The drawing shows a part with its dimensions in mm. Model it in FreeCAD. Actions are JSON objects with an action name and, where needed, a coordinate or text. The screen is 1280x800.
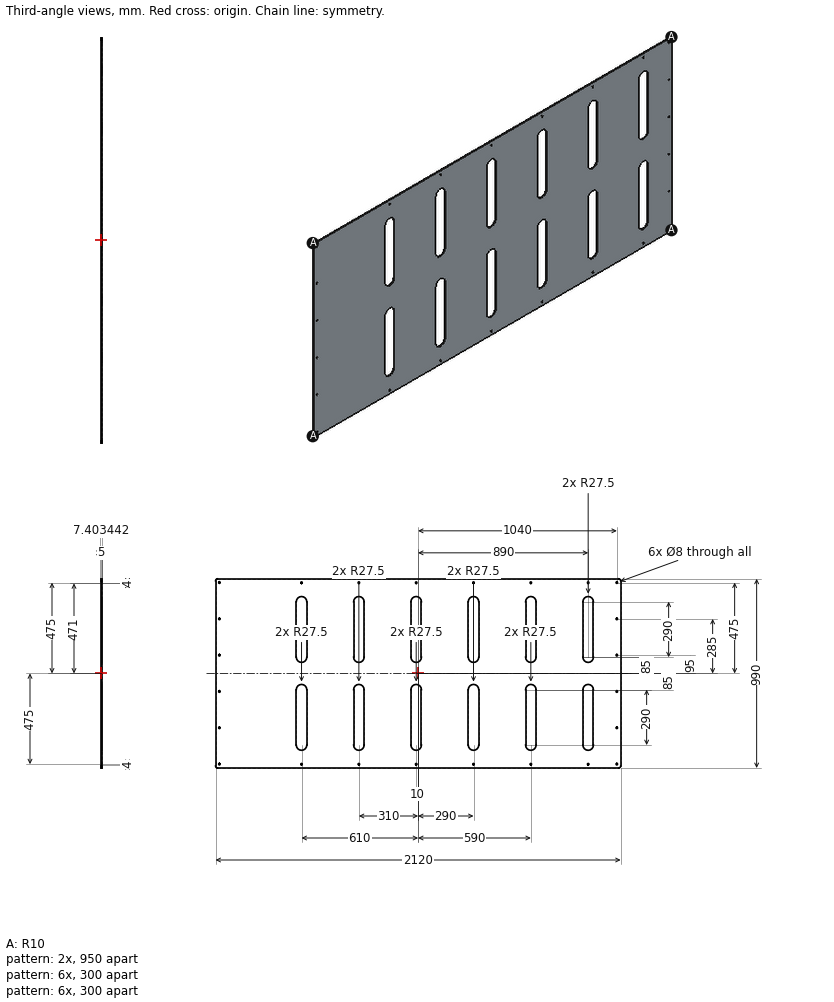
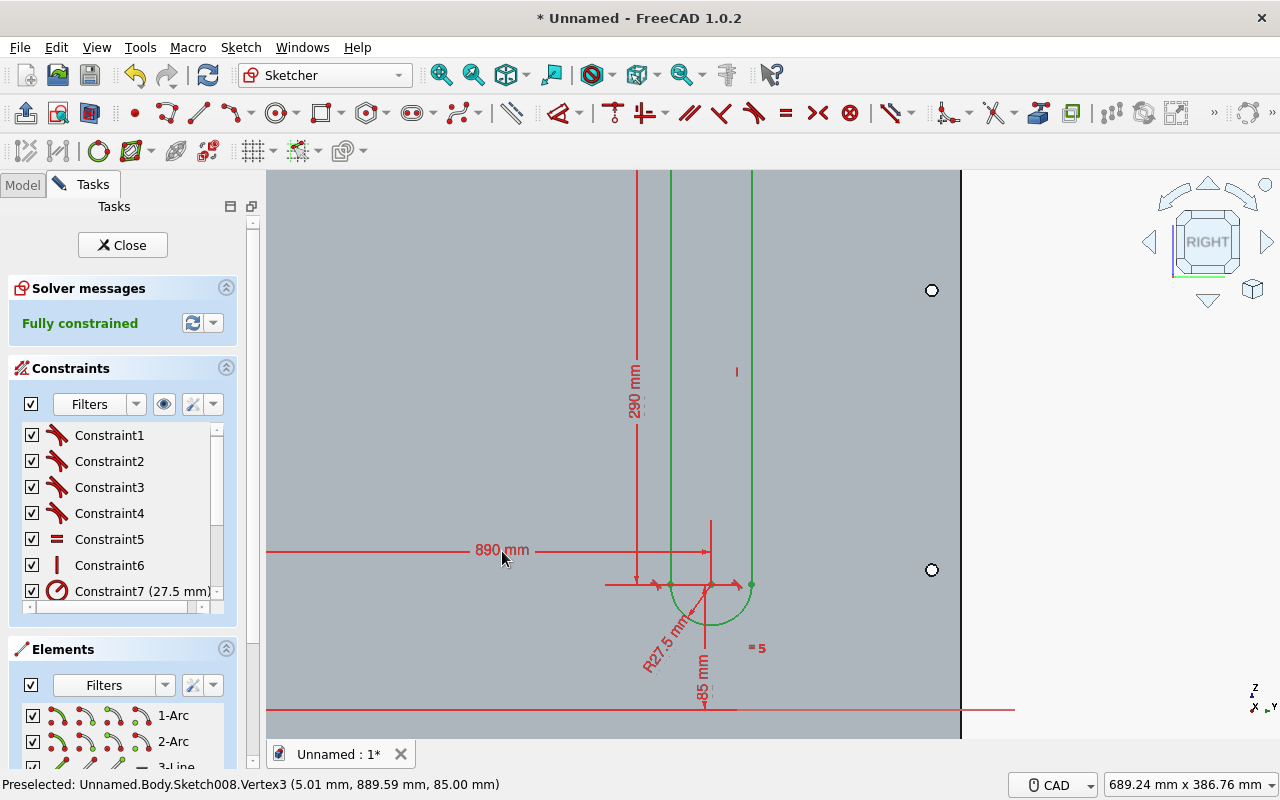
{"action": "left_click", "coordinate": [123, 245]}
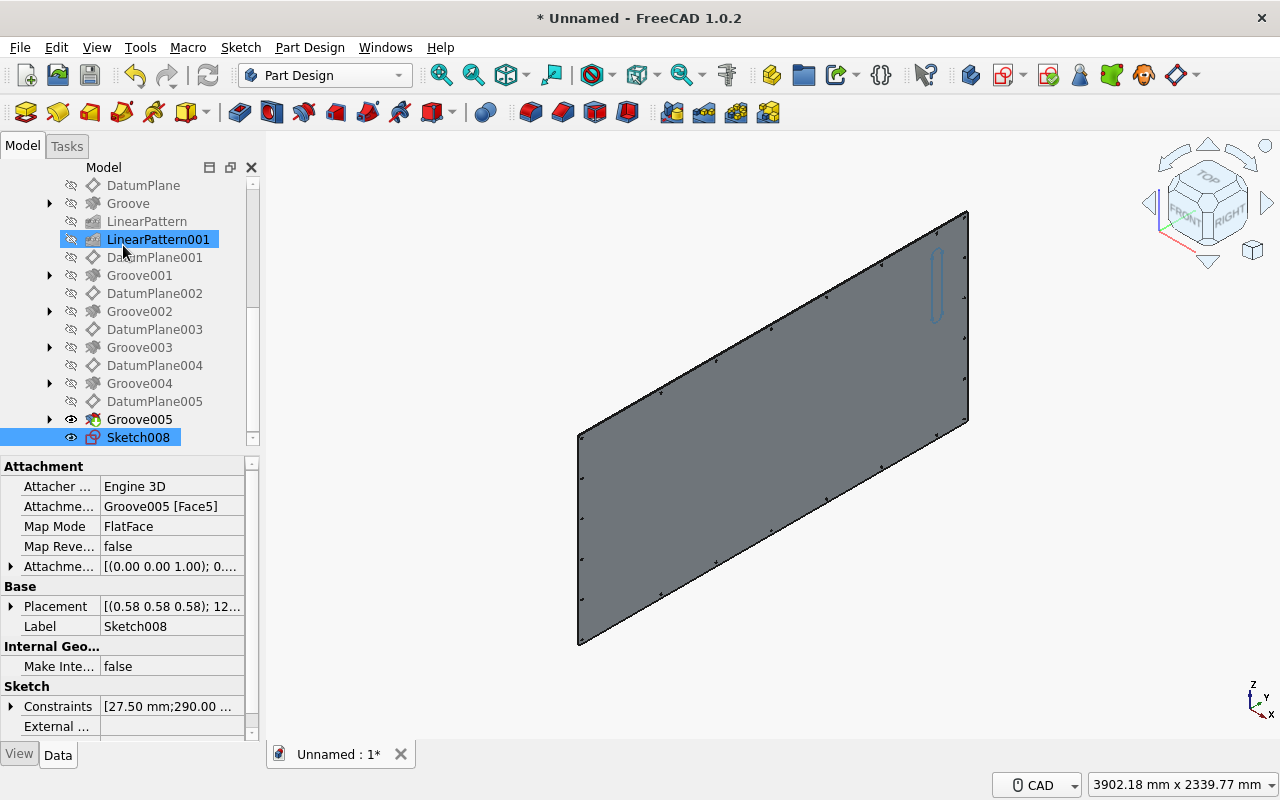
{"action": "left_click", "coordinate": [240, 112]}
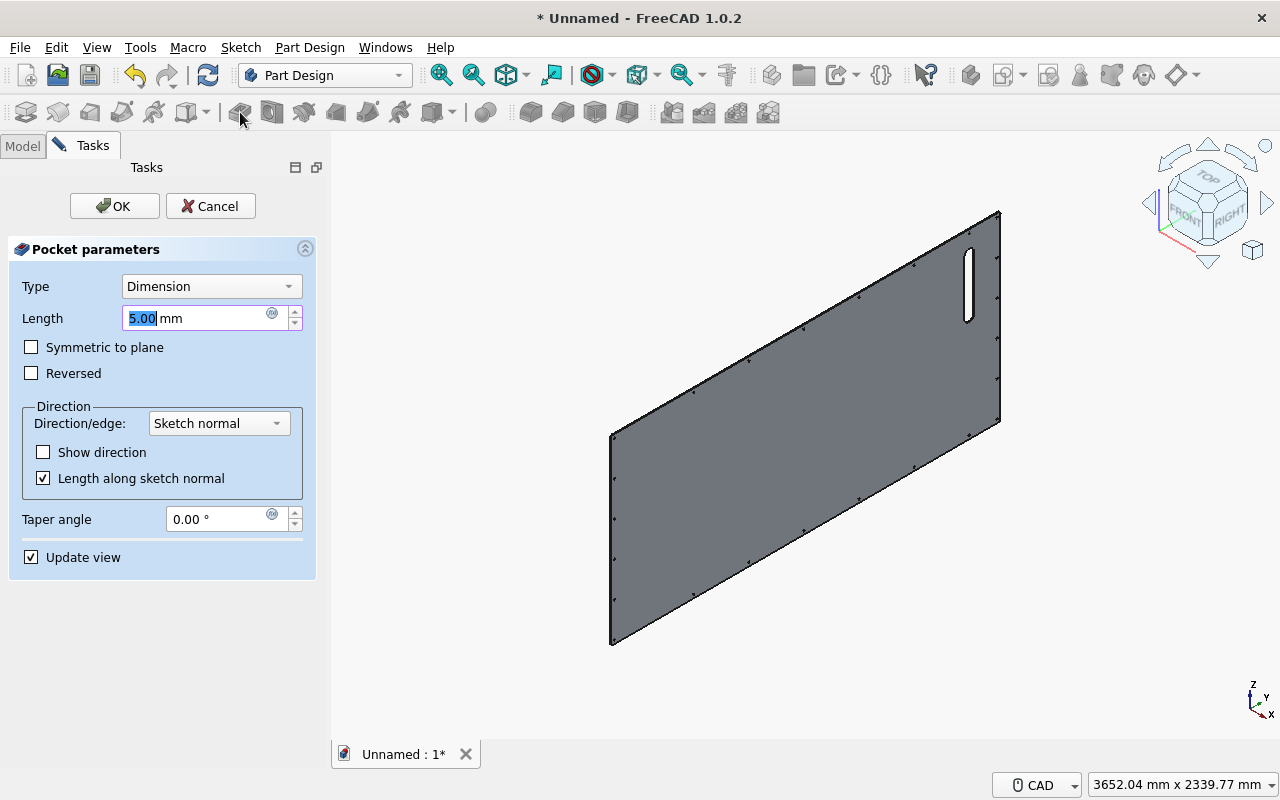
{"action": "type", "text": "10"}
{"action": "key", "text": "Tab"}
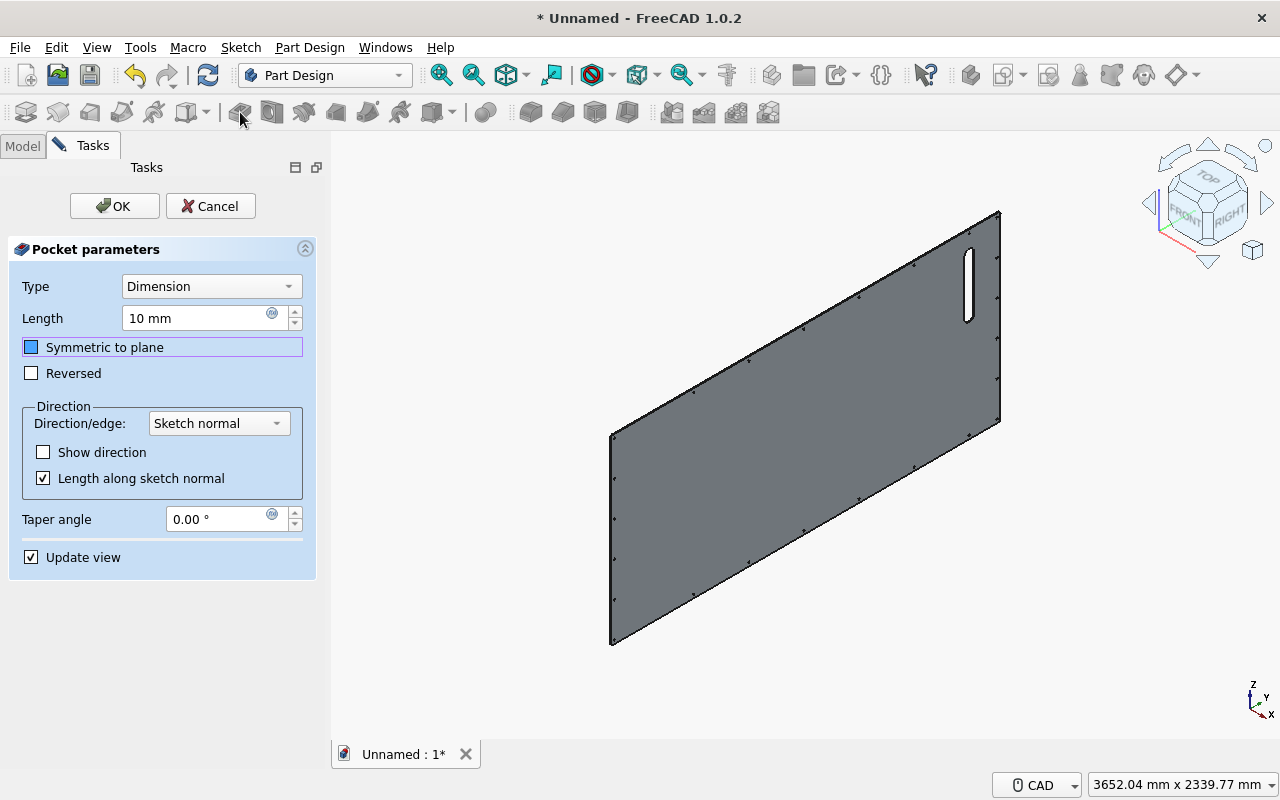
{"action": "left_click", "coordinate": [115, 206]}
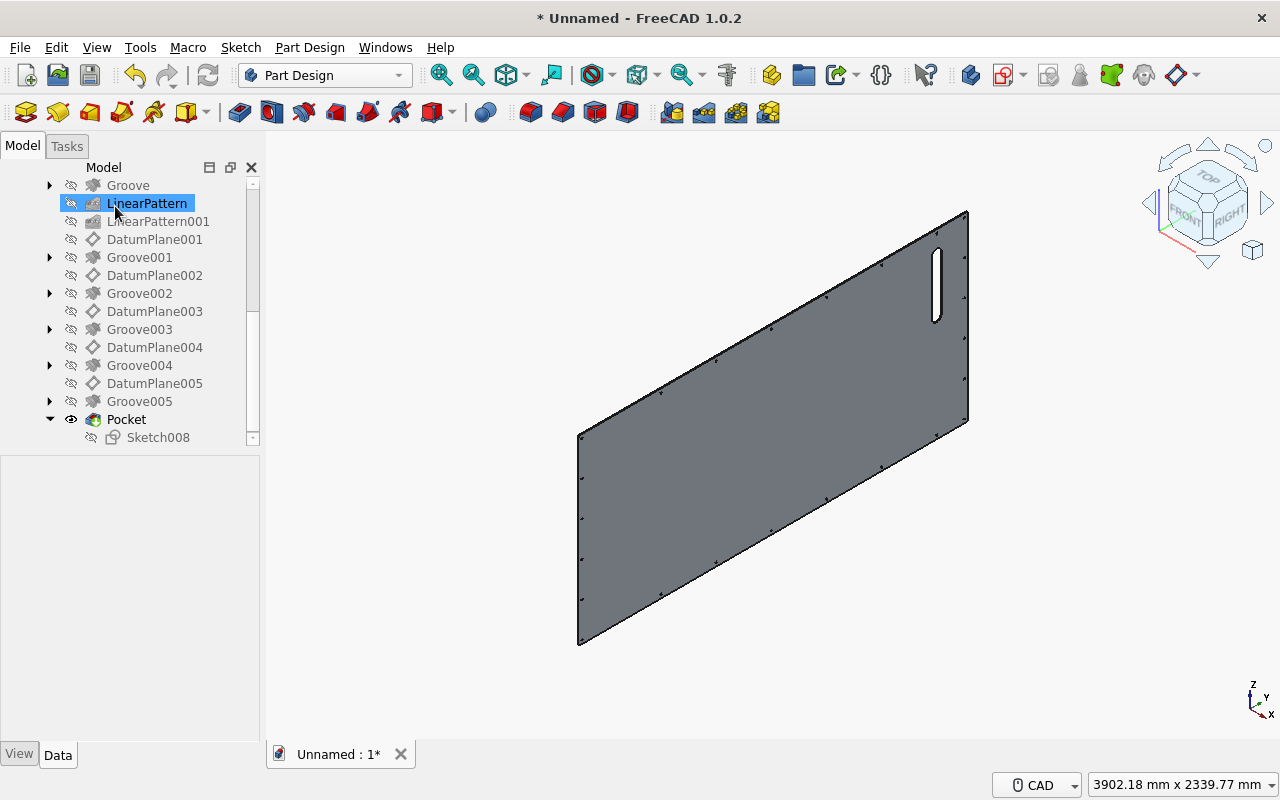
{"action": "left_click", "coordinate": [116, 419]}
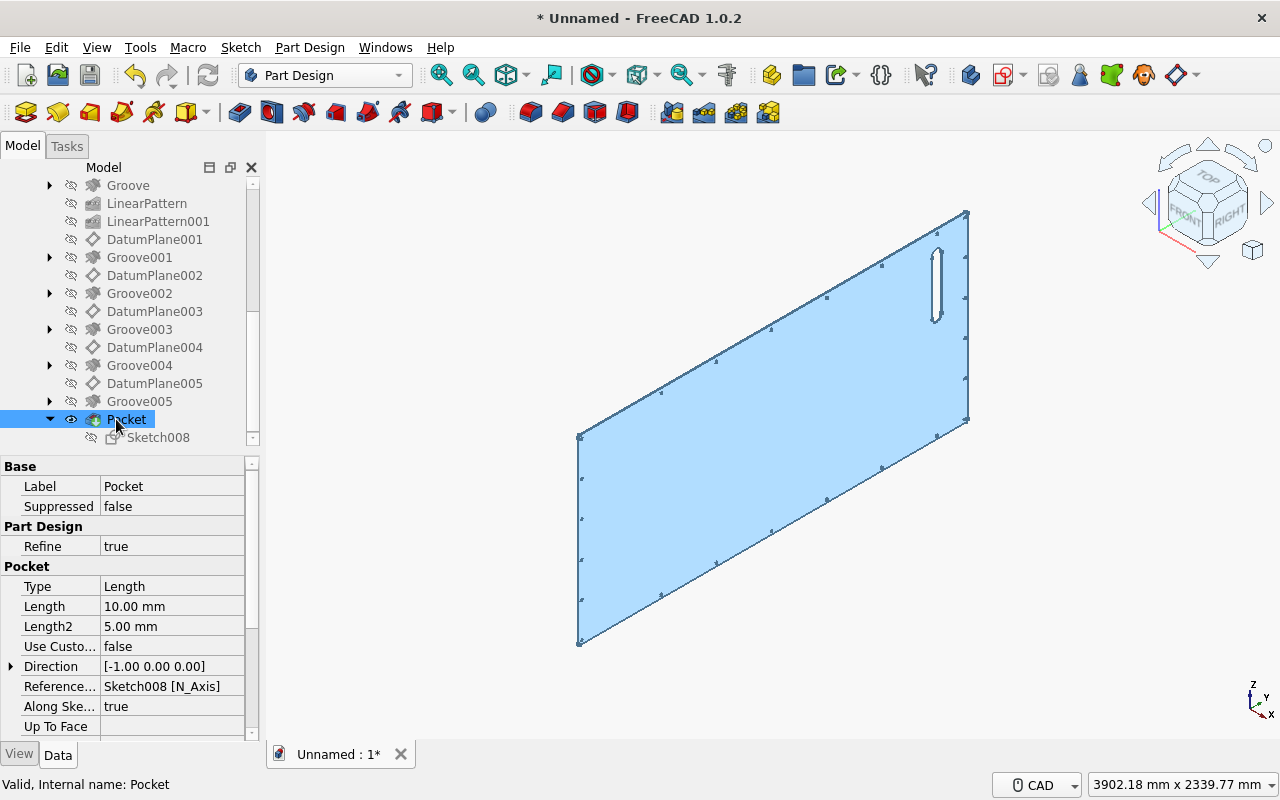
{"action": "left_click", "coordinate": [704, 112]}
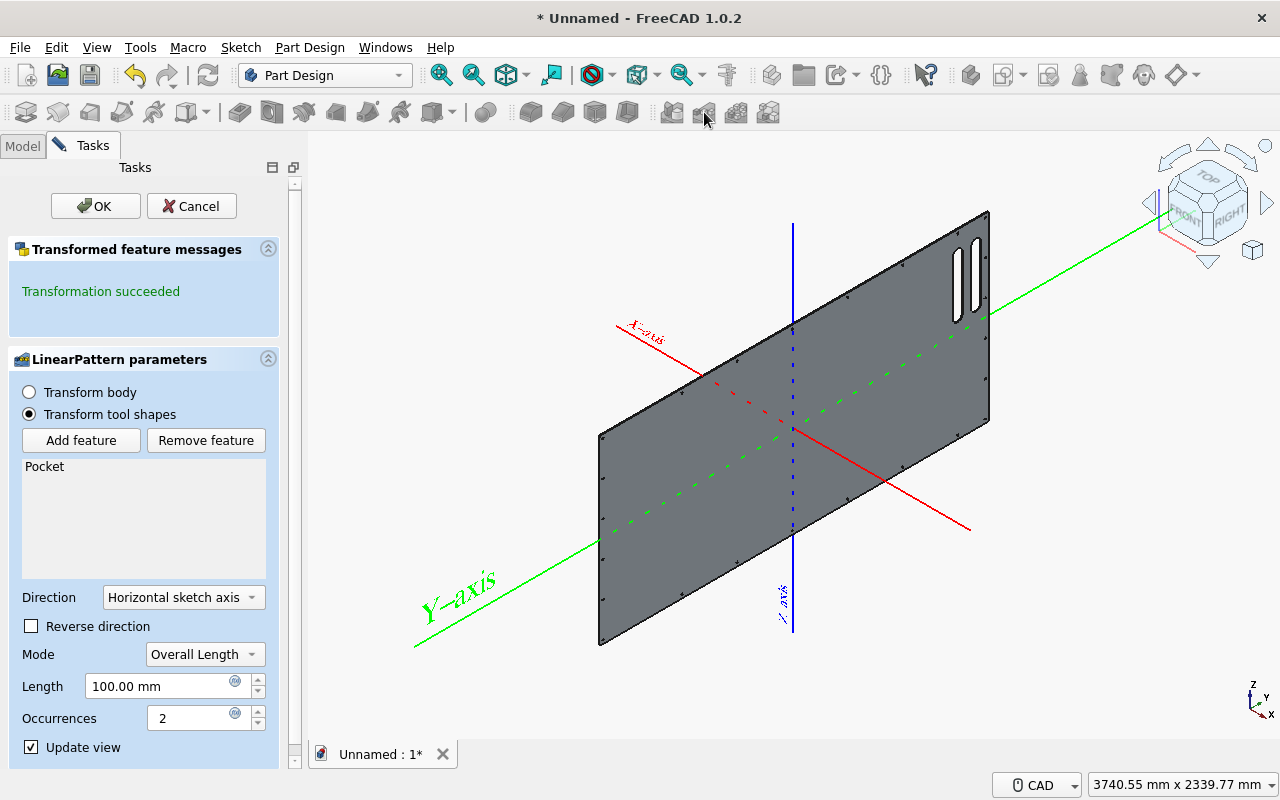
{"action": "left_click", "coordinate": [184, 598]}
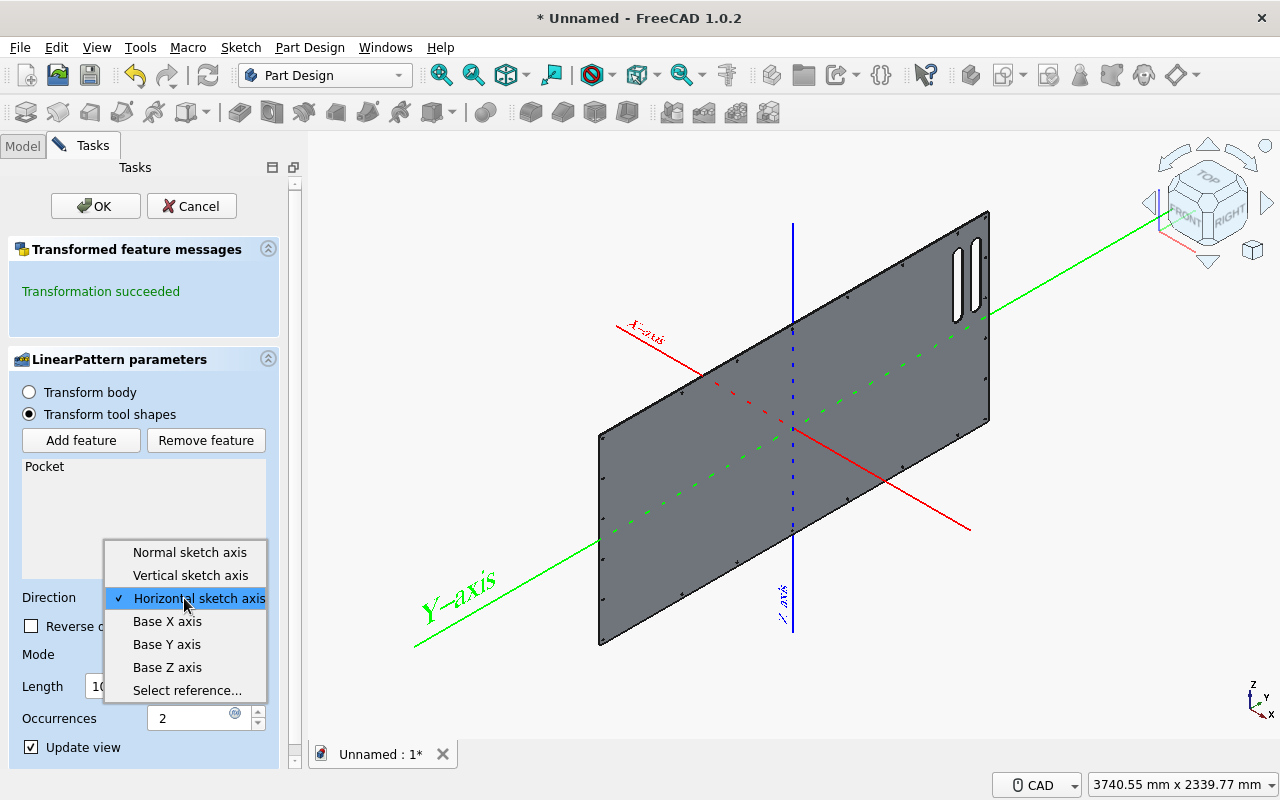
{"action": "left_click", "coordinate": [184, 644]}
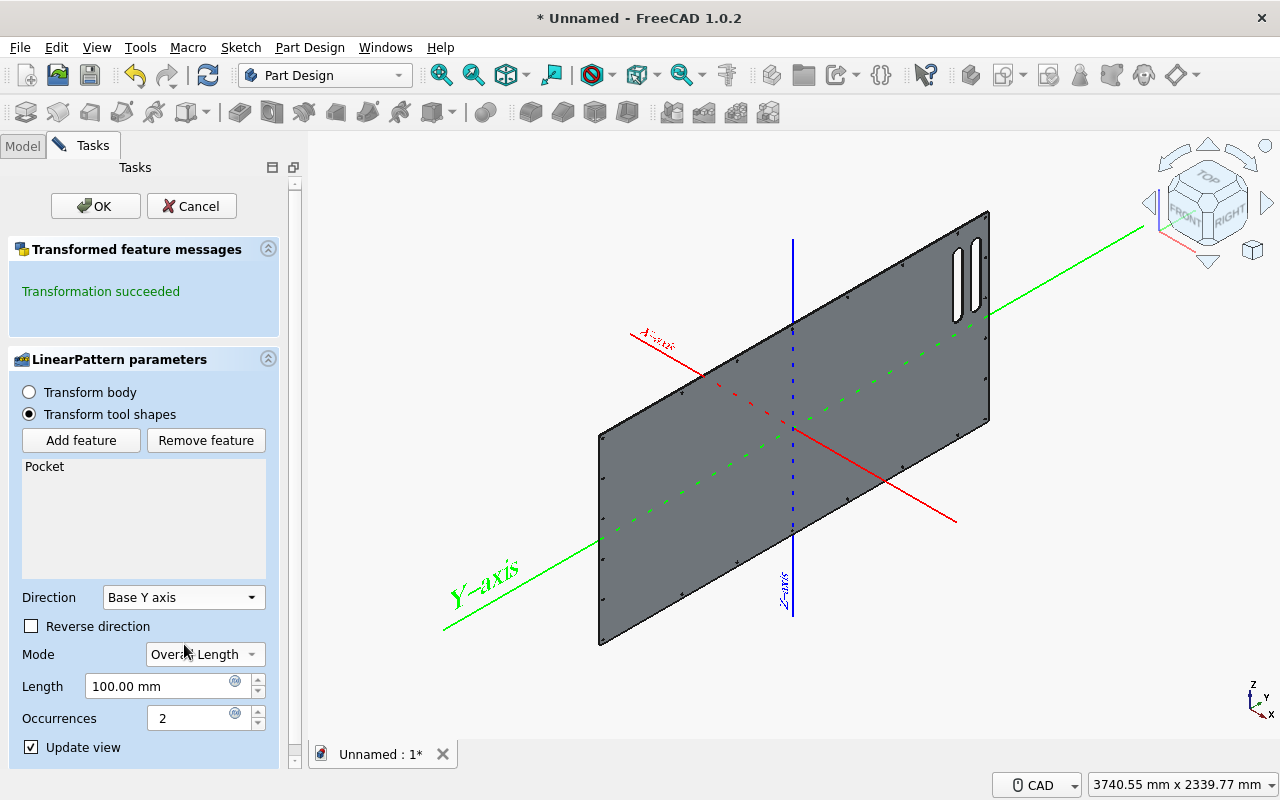
{"action": "left_click", "coordinate": [206, 654]}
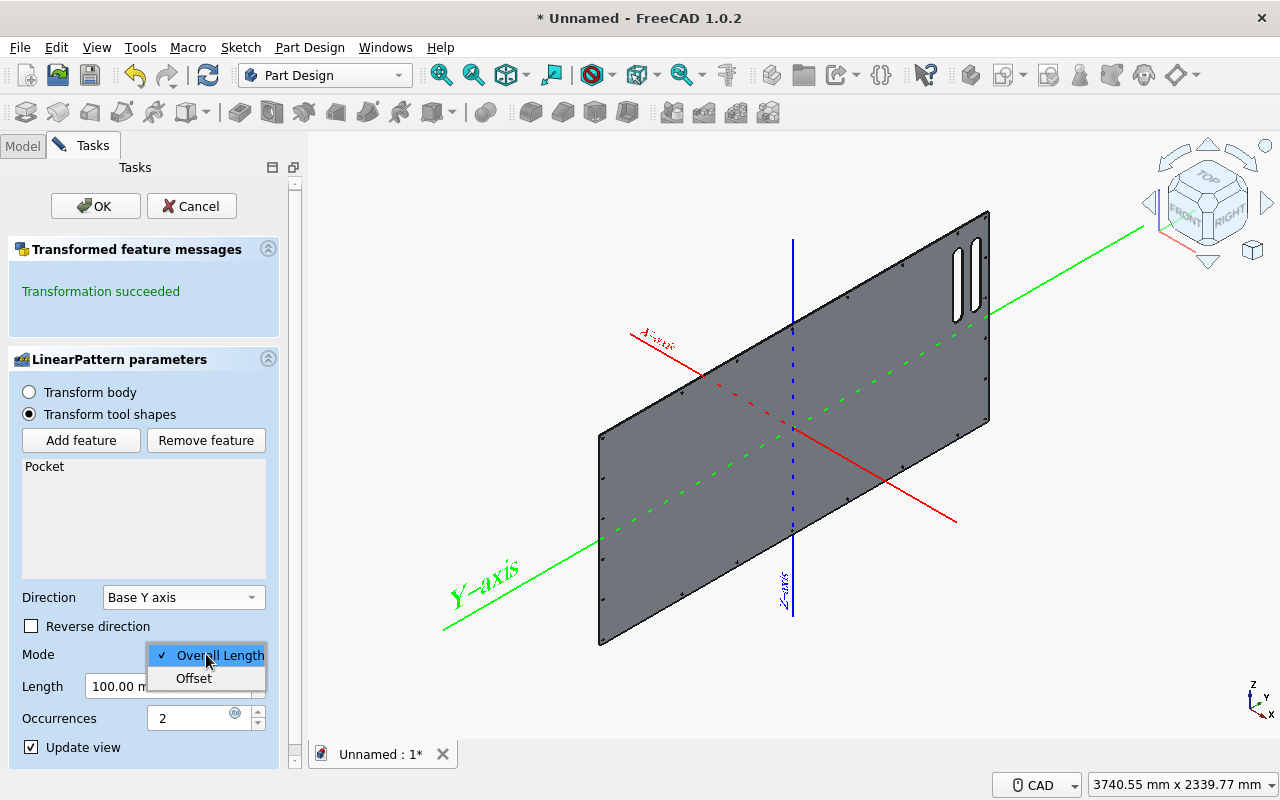
{"action": "left_click", "coordinate": [206, 678]}